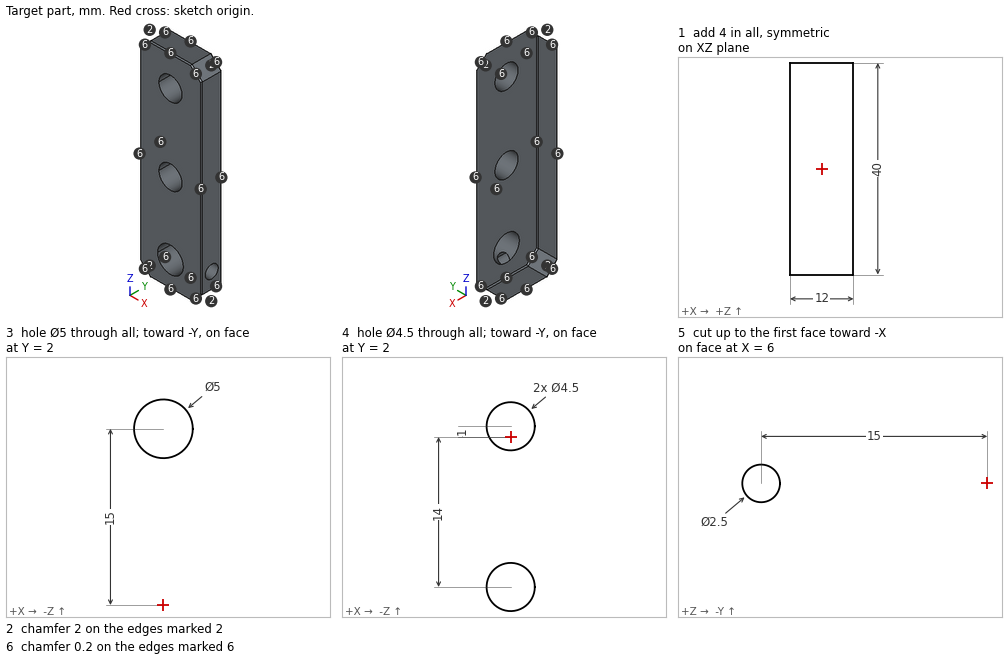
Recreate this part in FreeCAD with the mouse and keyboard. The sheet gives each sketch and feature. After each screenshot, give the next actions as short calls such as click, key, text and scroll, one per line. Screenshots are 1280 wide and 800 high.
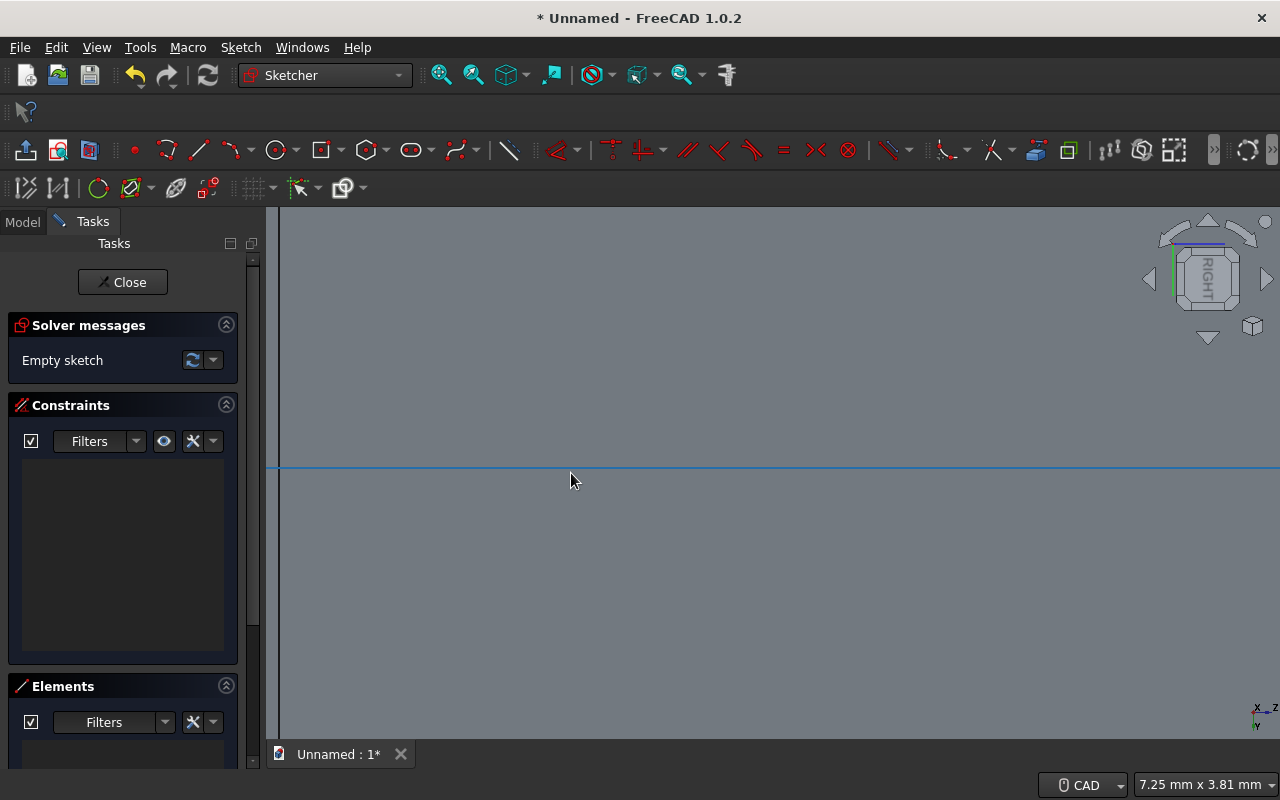
click(276, 150)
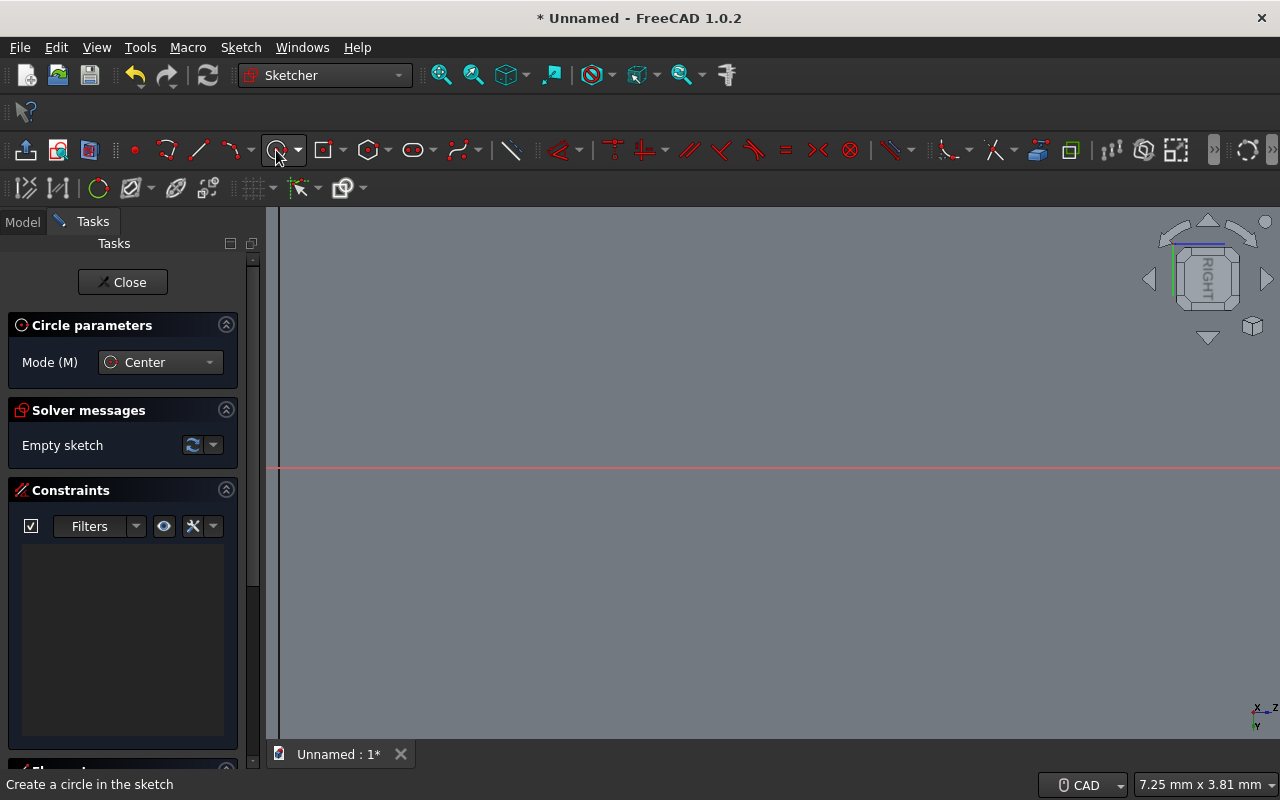
click(698, 468)
click(821, 344)
key(Escape)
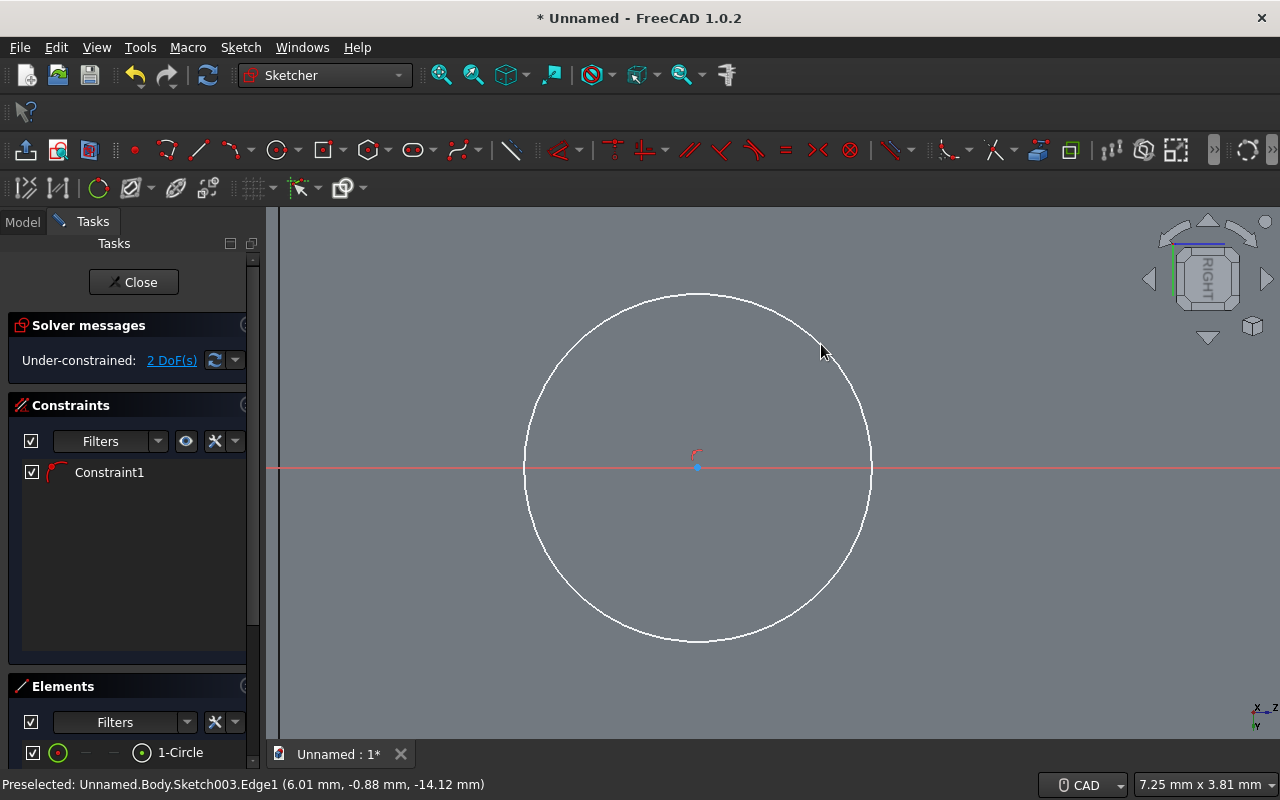
click(558, 150)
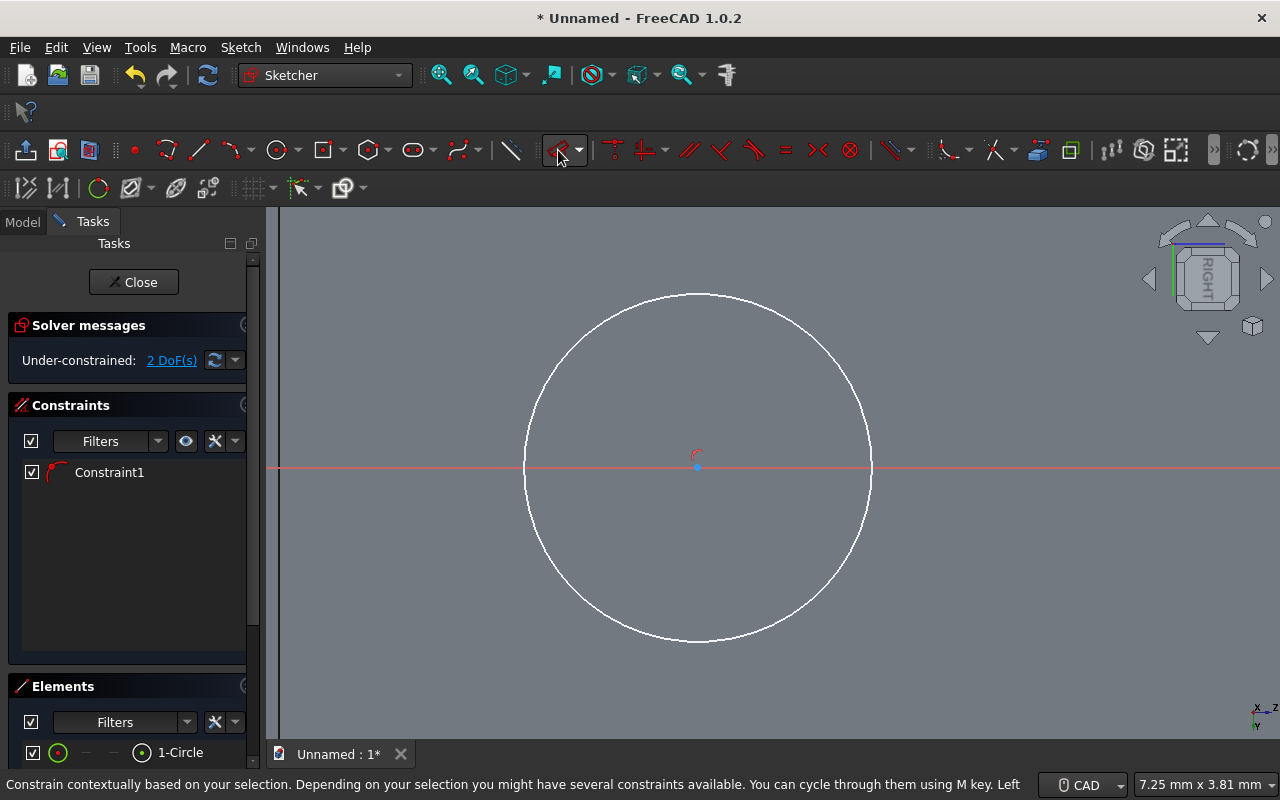
click(821, 345)
click(844, 322)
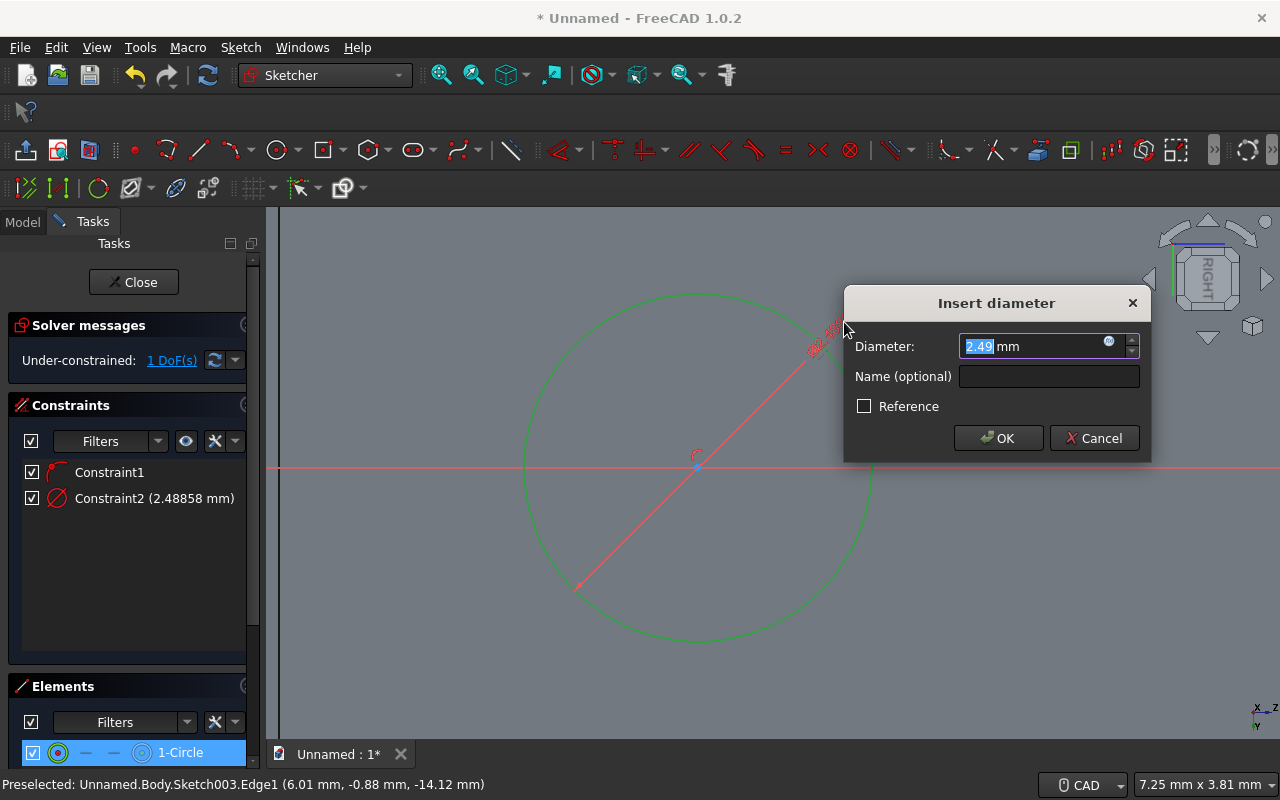
text(2.5)
key(Return)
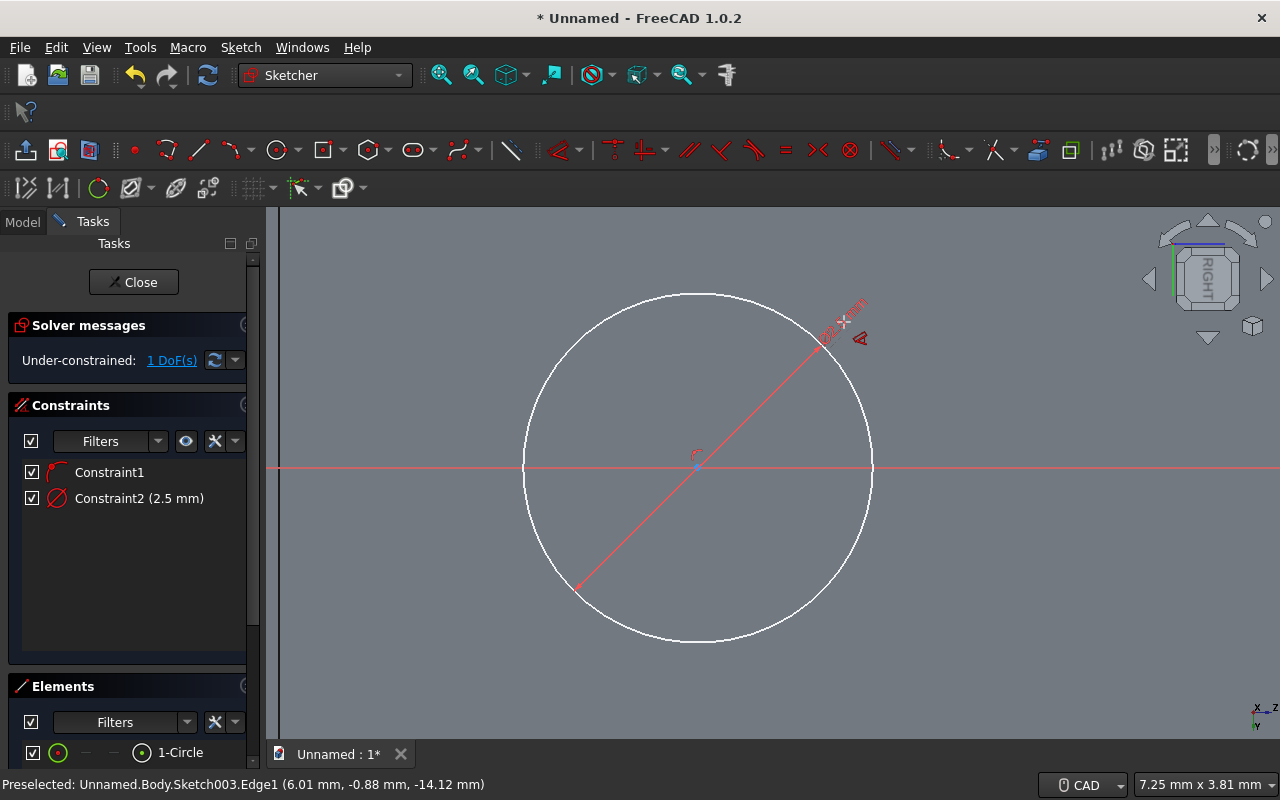
click(698, 468)
click(907, 502)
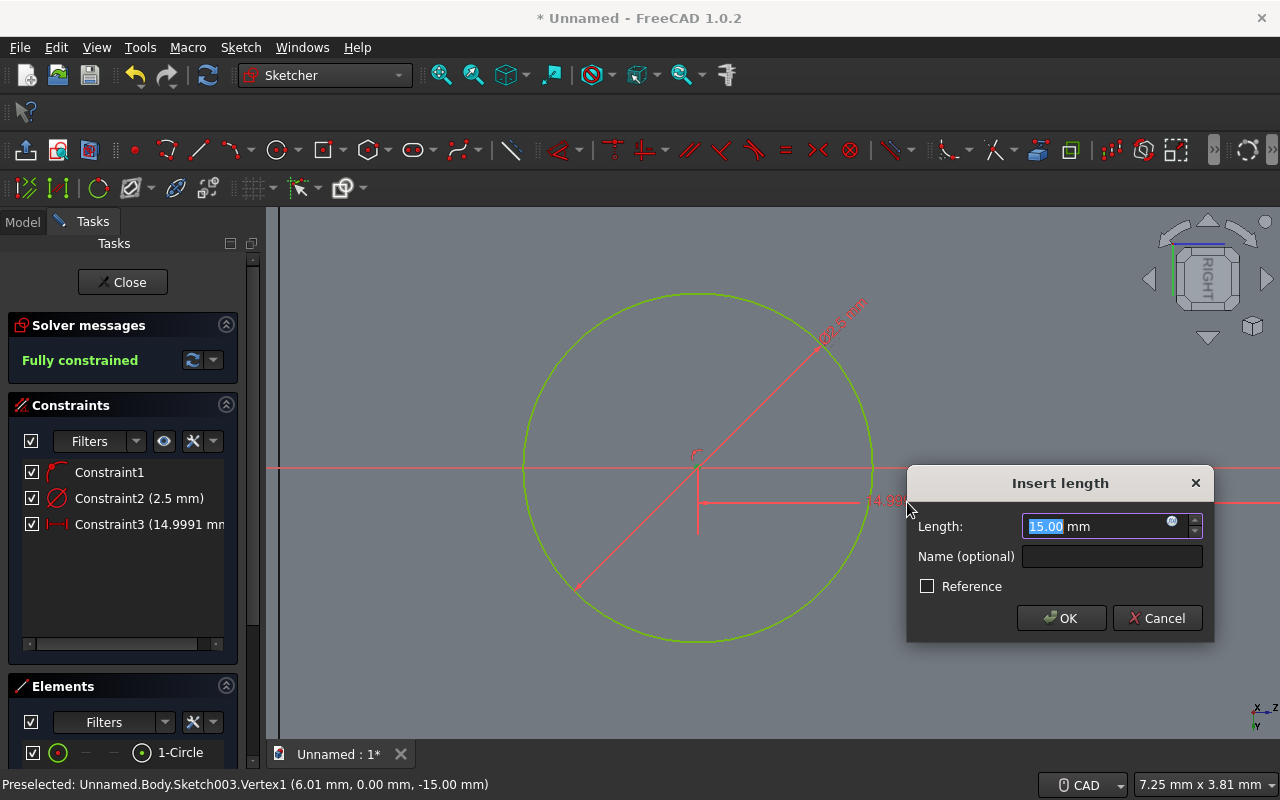
text(15)
key(Return)
key(Escape)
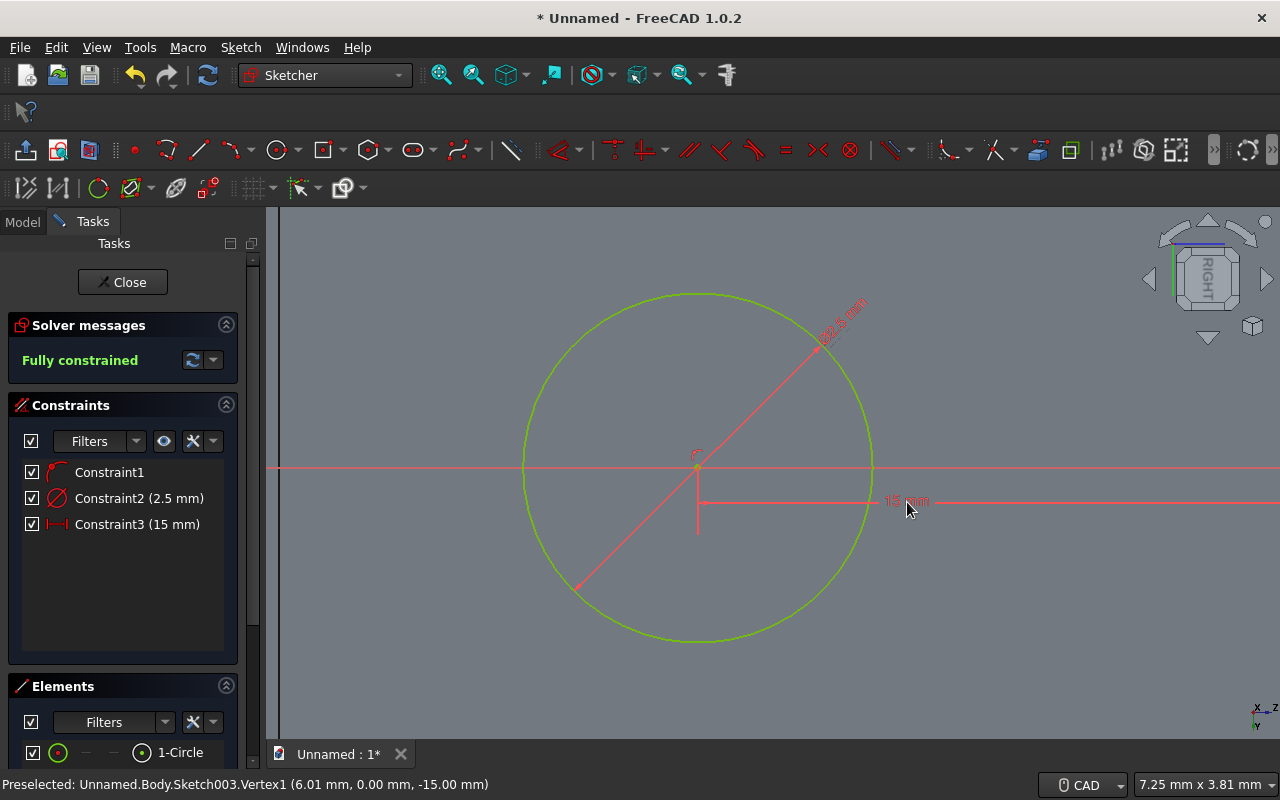
click(123, 282)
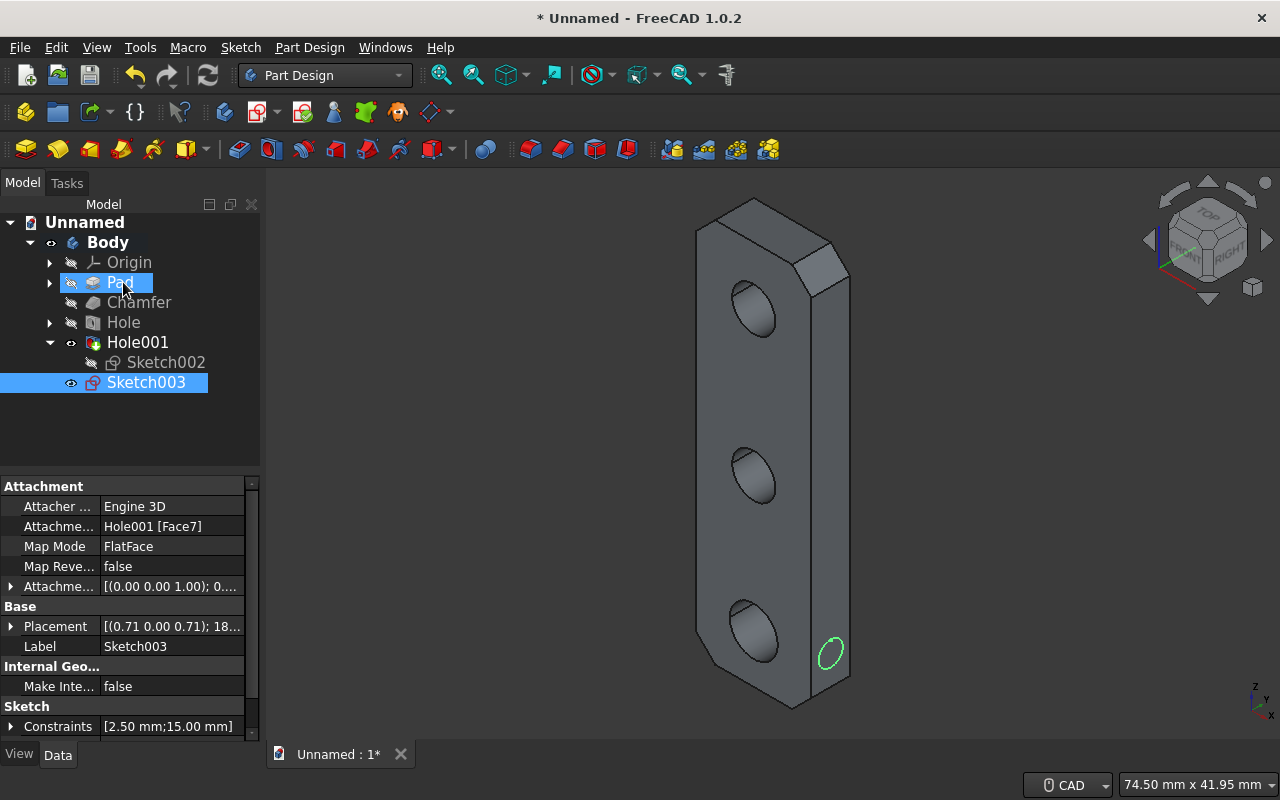
click(240, 150)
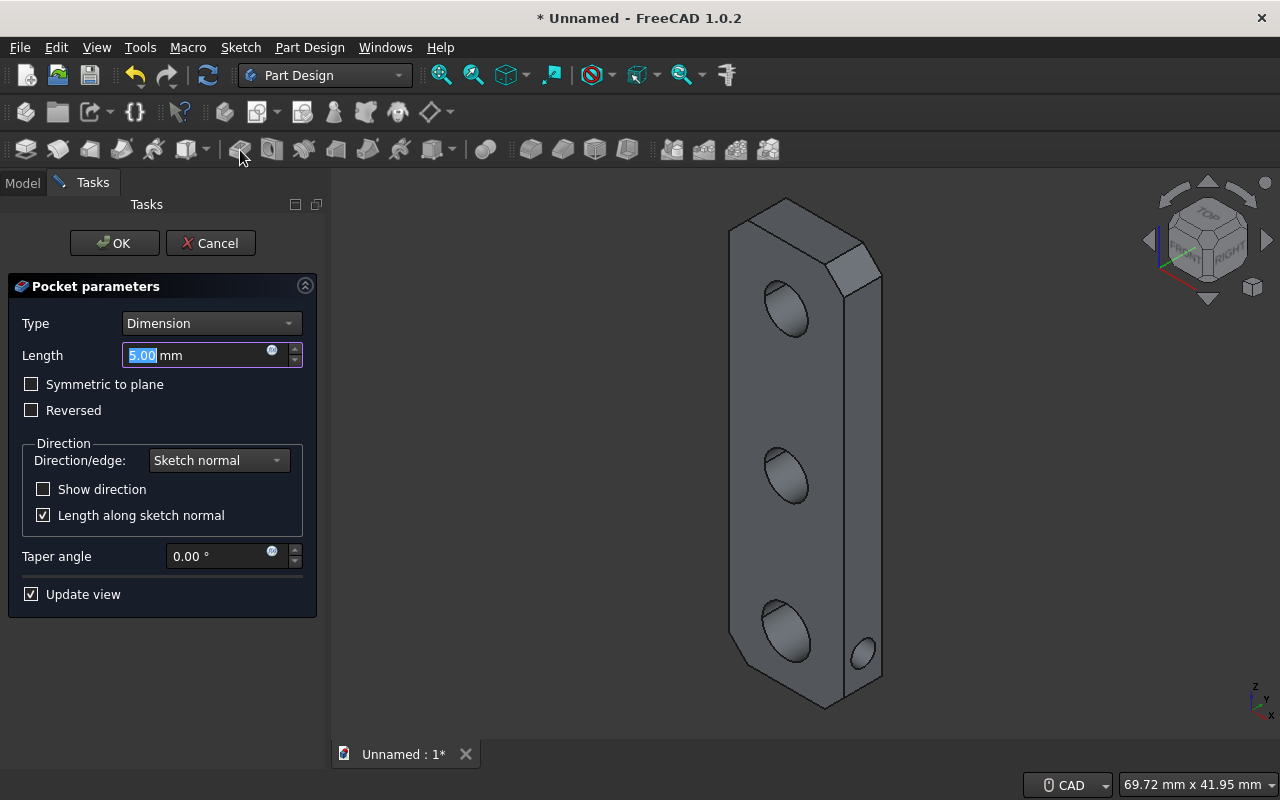
click(212, 324)